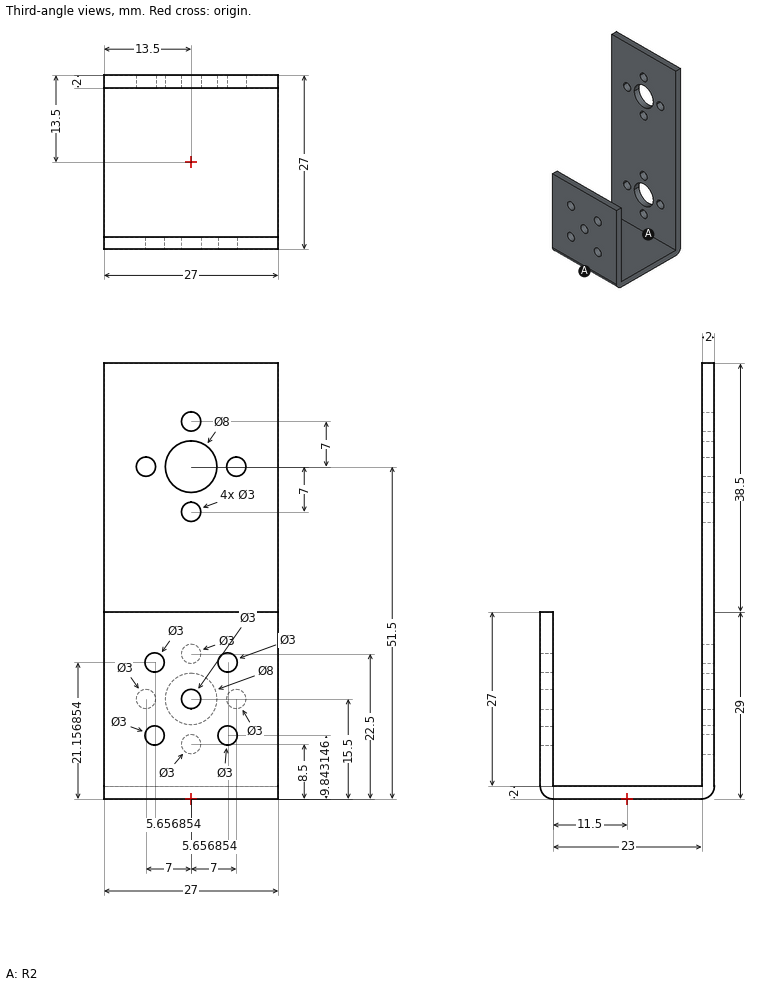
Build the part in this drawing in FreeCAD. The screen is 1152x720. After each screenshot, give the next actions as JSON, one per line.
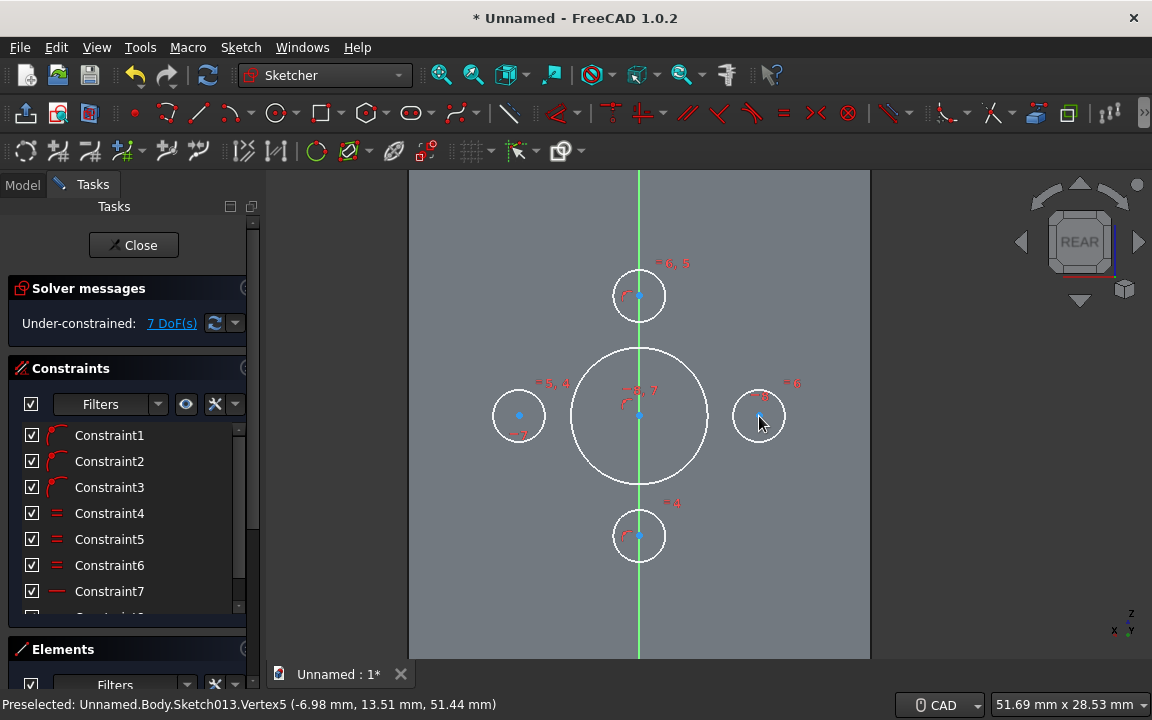
{"action": "left_click", "coordinate": [556, 114]}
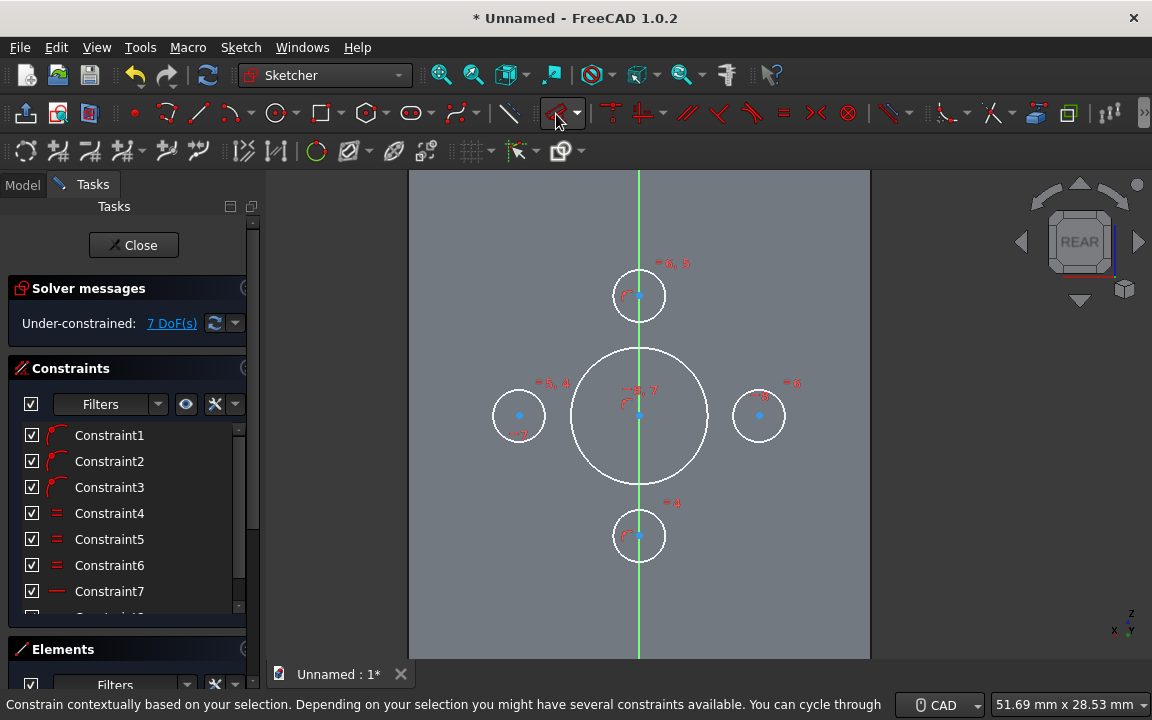
{"action": "left_click", "coordinate": [688, 368]}
{"action": "left_click", "coordinate": [711, 346]}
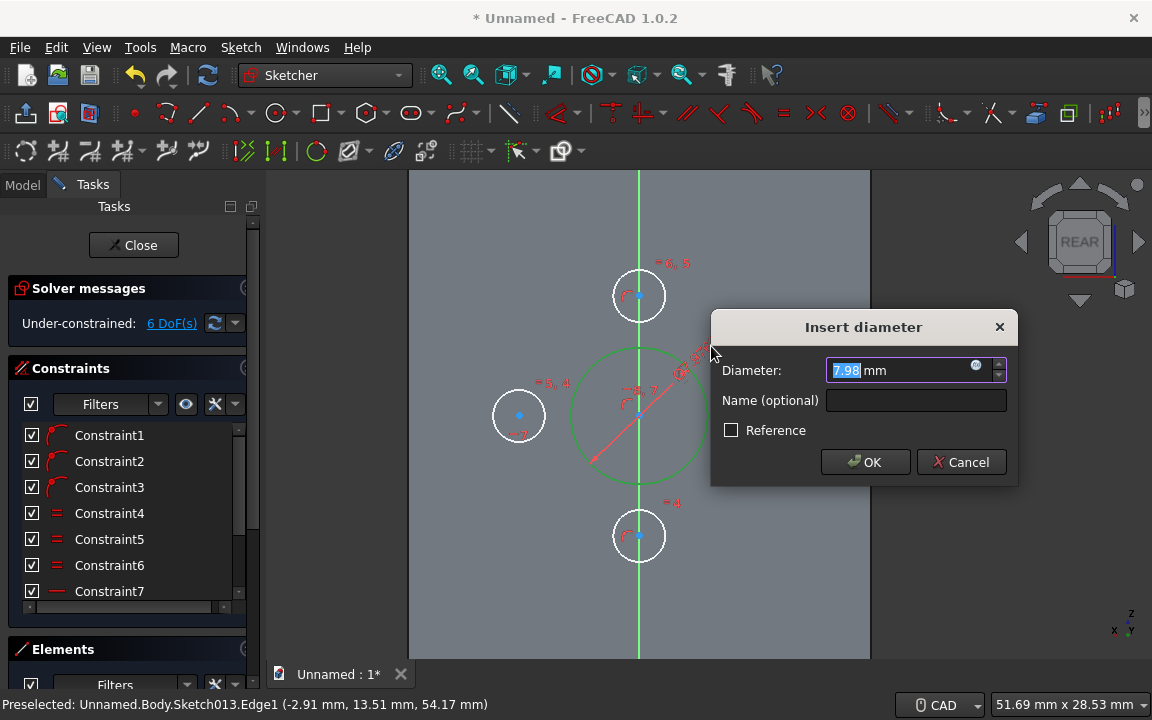
{"action": "type", "text": "8"}
{"action": "key", "text": "Return"}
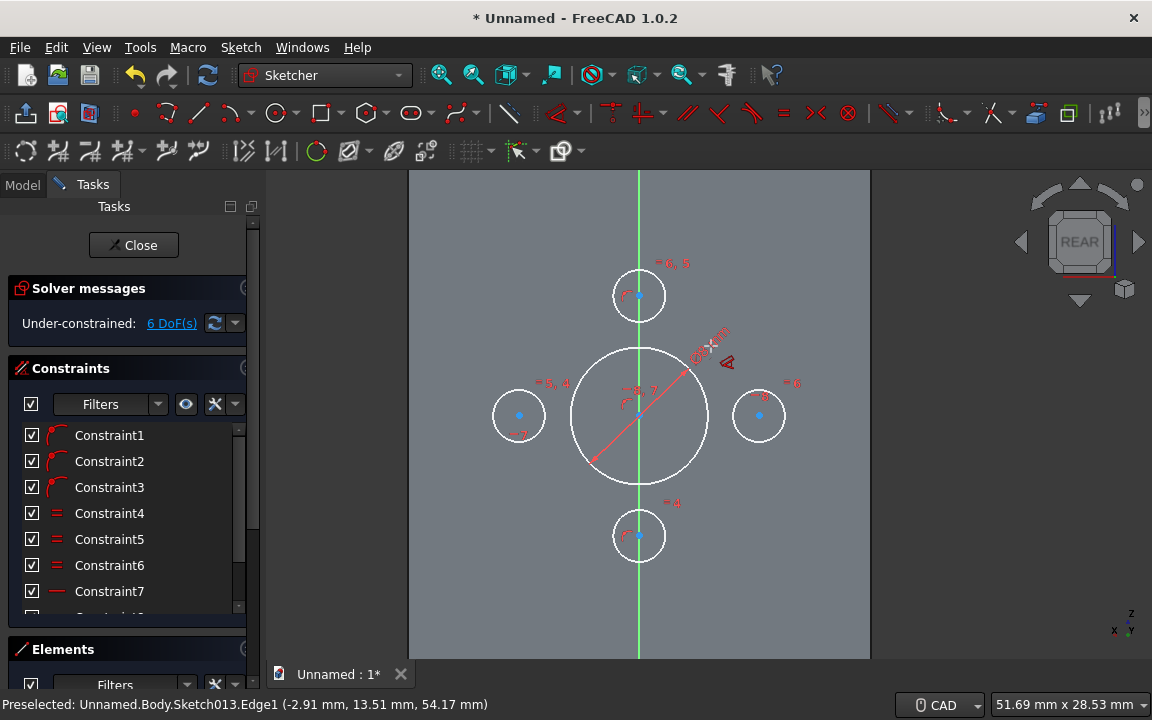
{"action": "left_click", "coordinate": [658, 518]}
{"action": "left_click", "coordinate": [681, 496]}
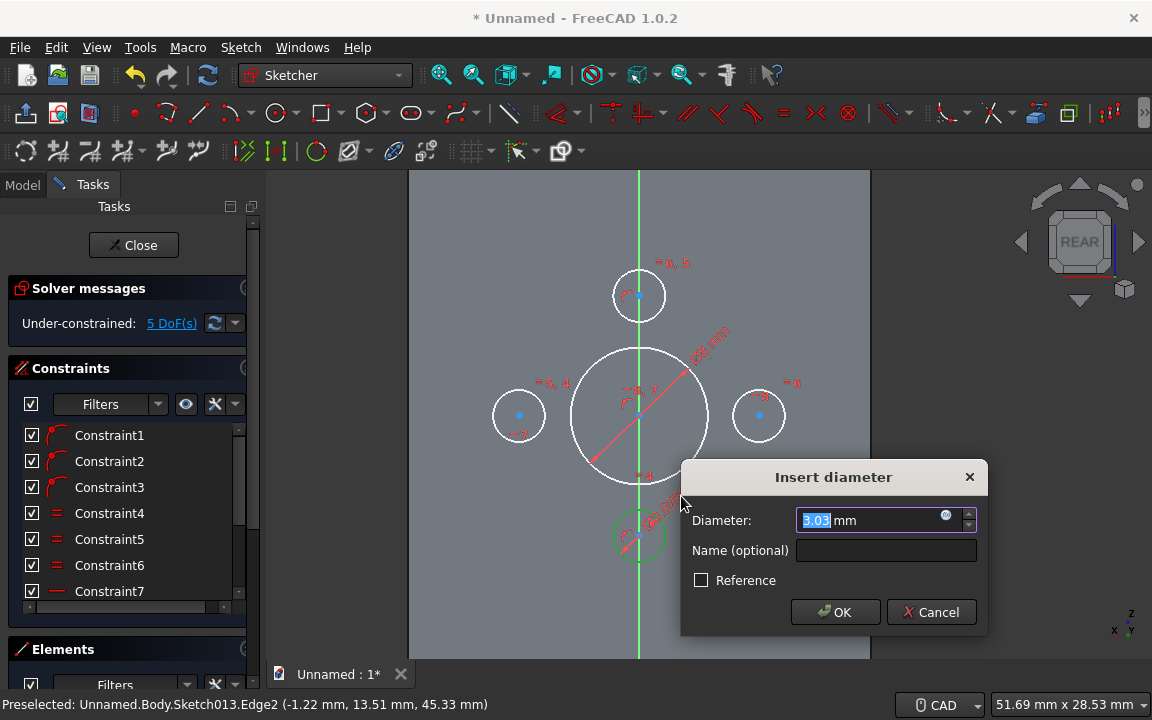
{"action": "type", "text": "3"}
{"action": "key", "text": "Return"}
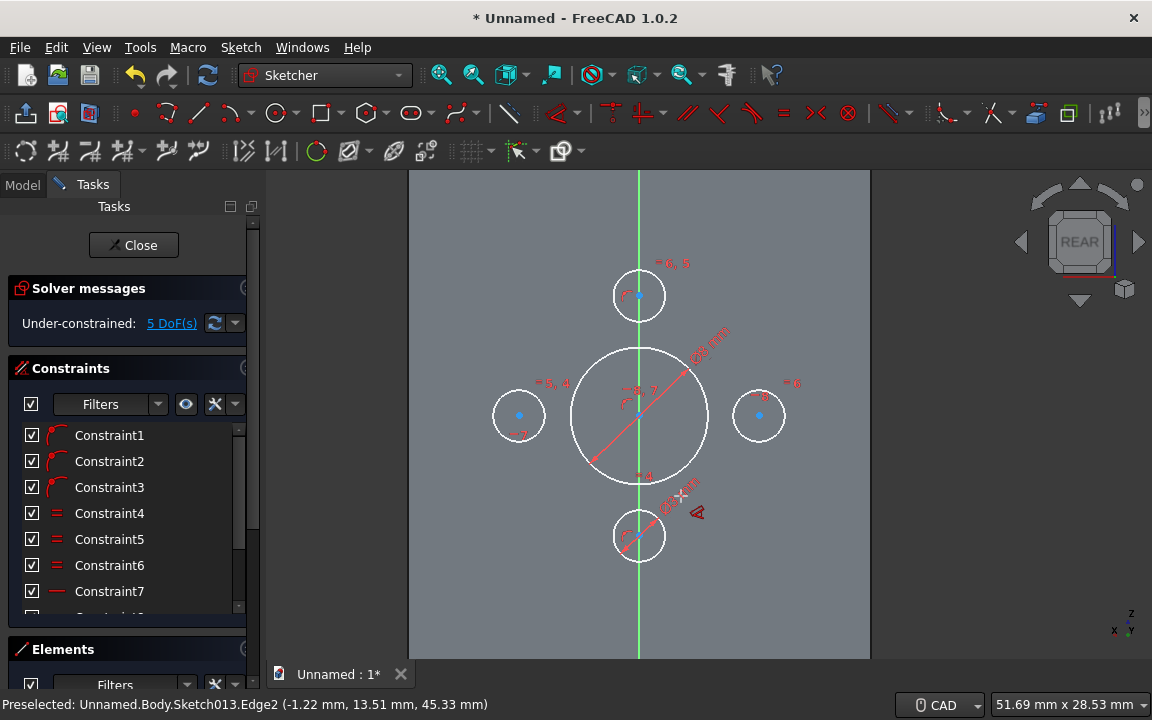
{"action": "left_click", "coordinate": [519, 416]}
{"action": "left_click", "coordinate": [551, 382]}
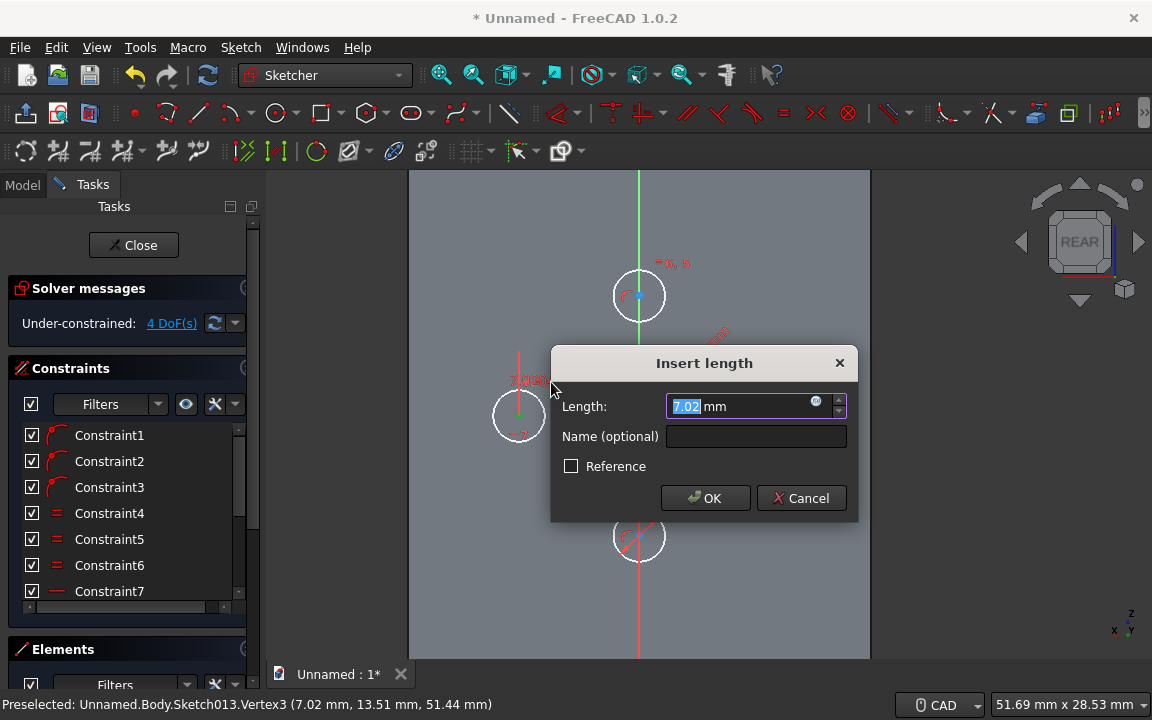
{"action": "type", "text": "7"}
{"action": "key", "text": "Return"}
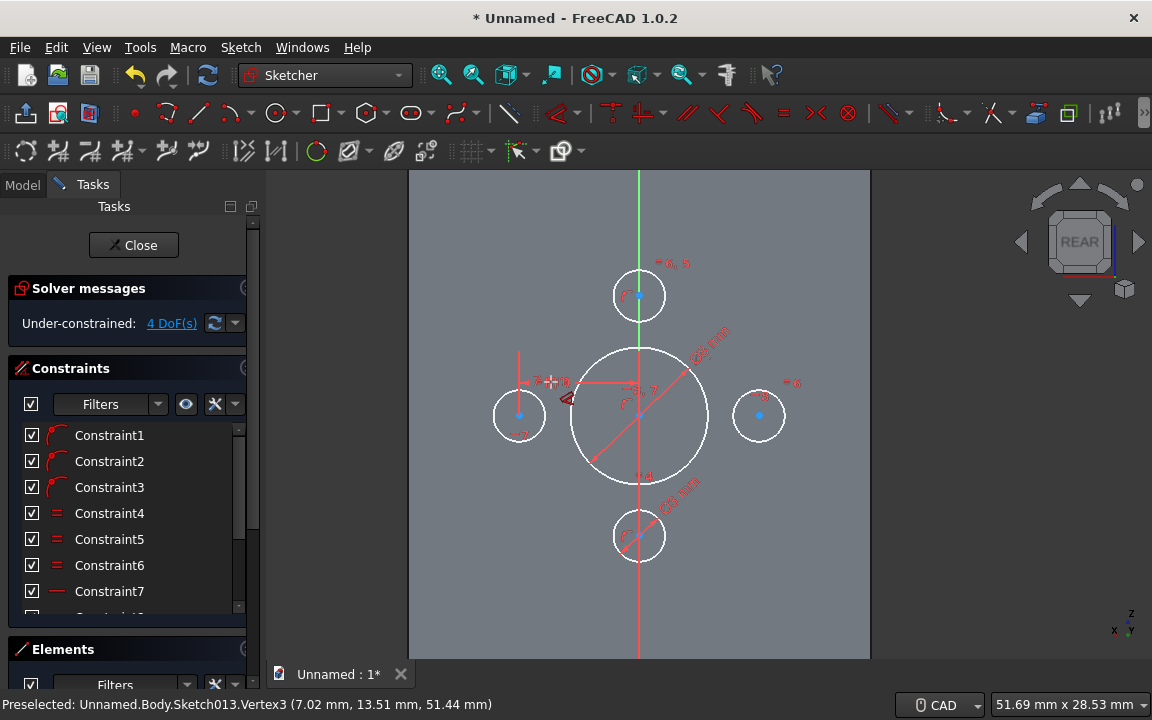
{"action": "left_click", "coordinate": [759, 416]}
{"action": "left_click", "coordinate": [672, 382]}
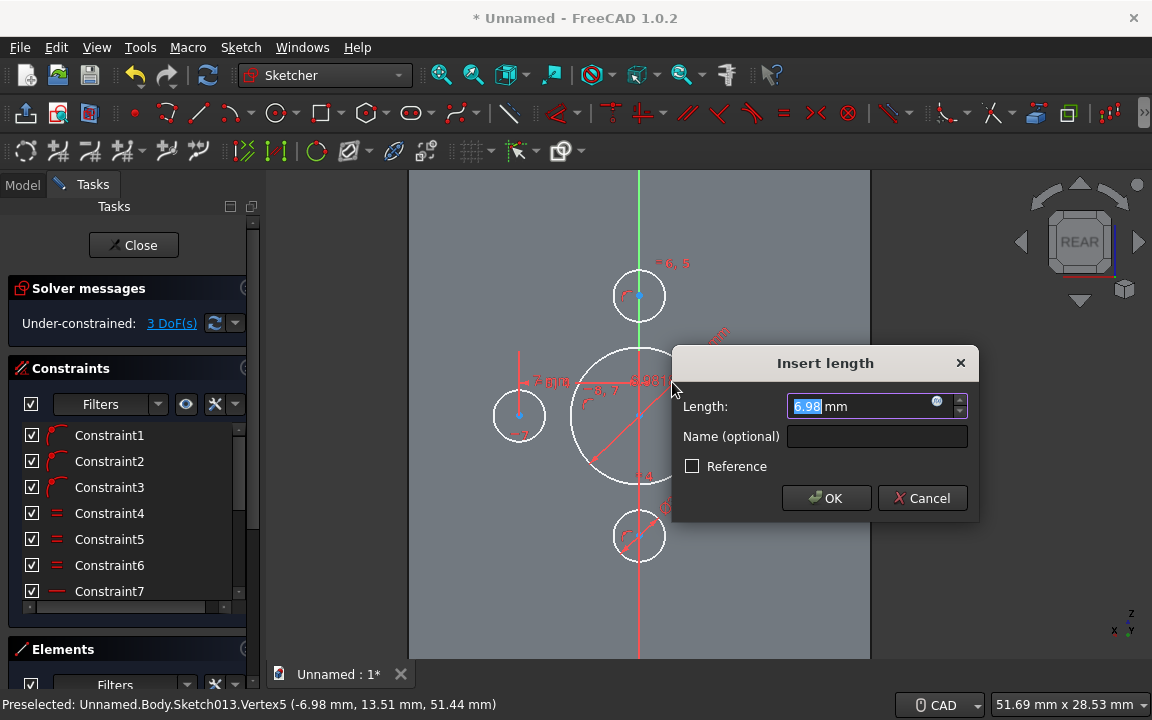
{"action": "type", "text": "7"}
{"action": "key", "text": "Return"}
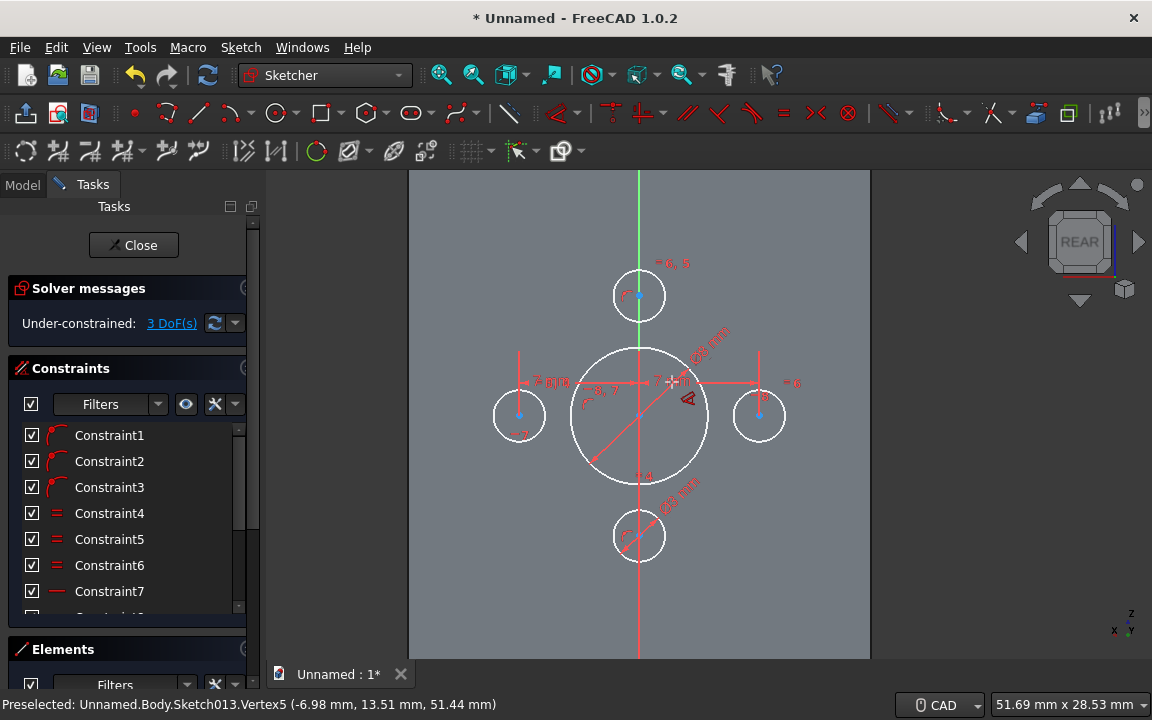
{"action": "left_click", "coordinate": [639, 416]}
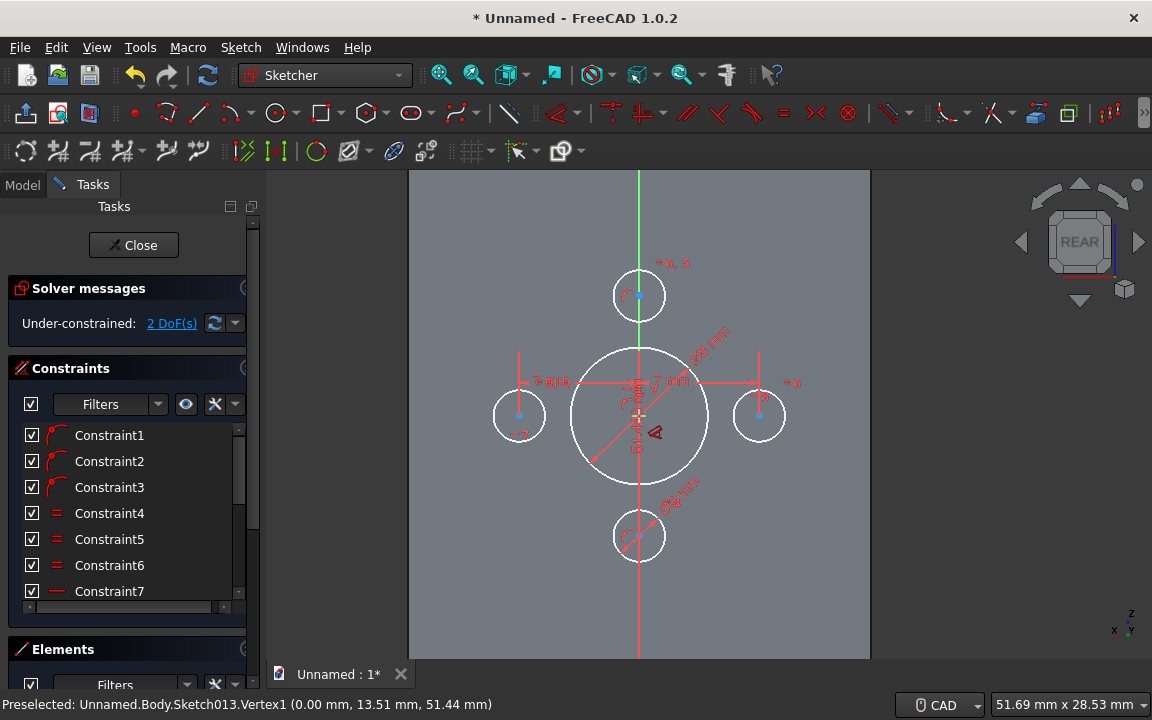
{"action": "left_click", "coordinate": [639, 536]}
{"action": "left_click", "coordinate": [673, 448]}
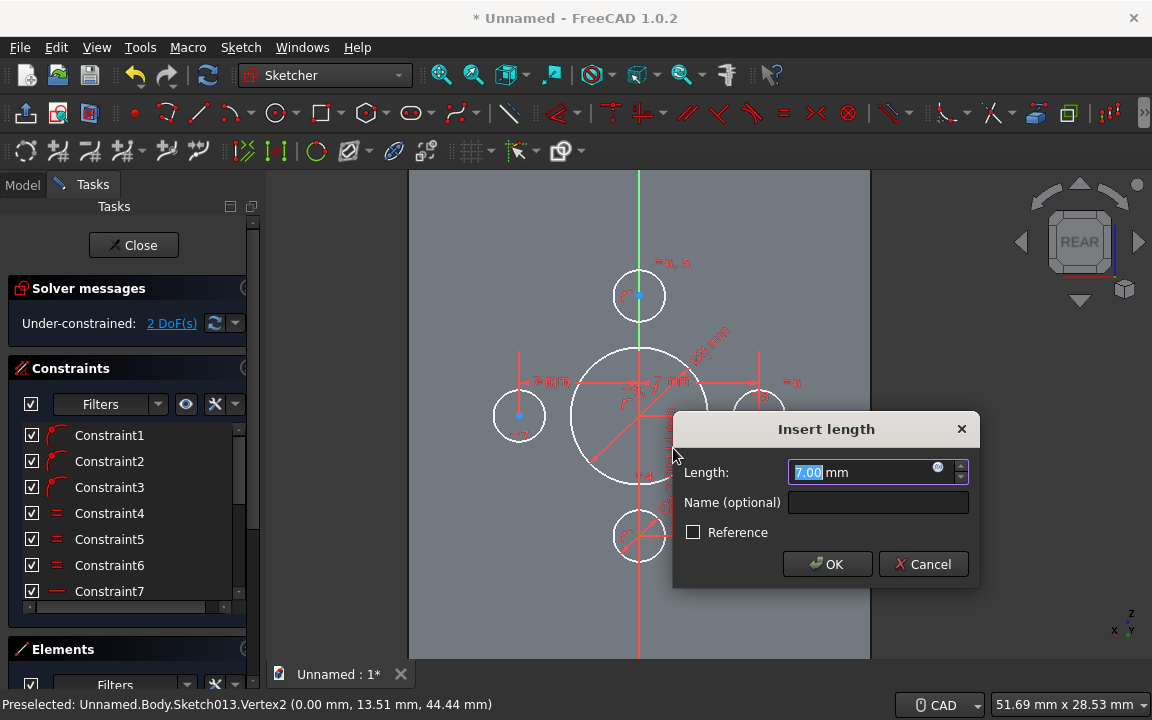
{"action": "type", "text": "7"}
{"action": "key", "text": "Return"}